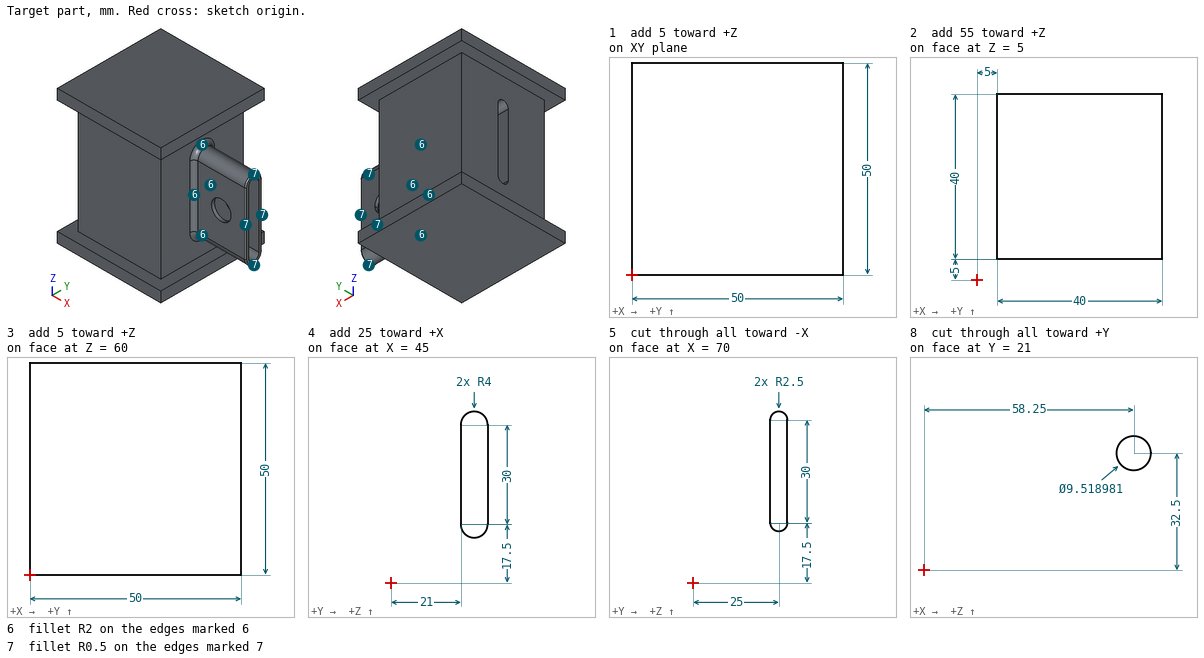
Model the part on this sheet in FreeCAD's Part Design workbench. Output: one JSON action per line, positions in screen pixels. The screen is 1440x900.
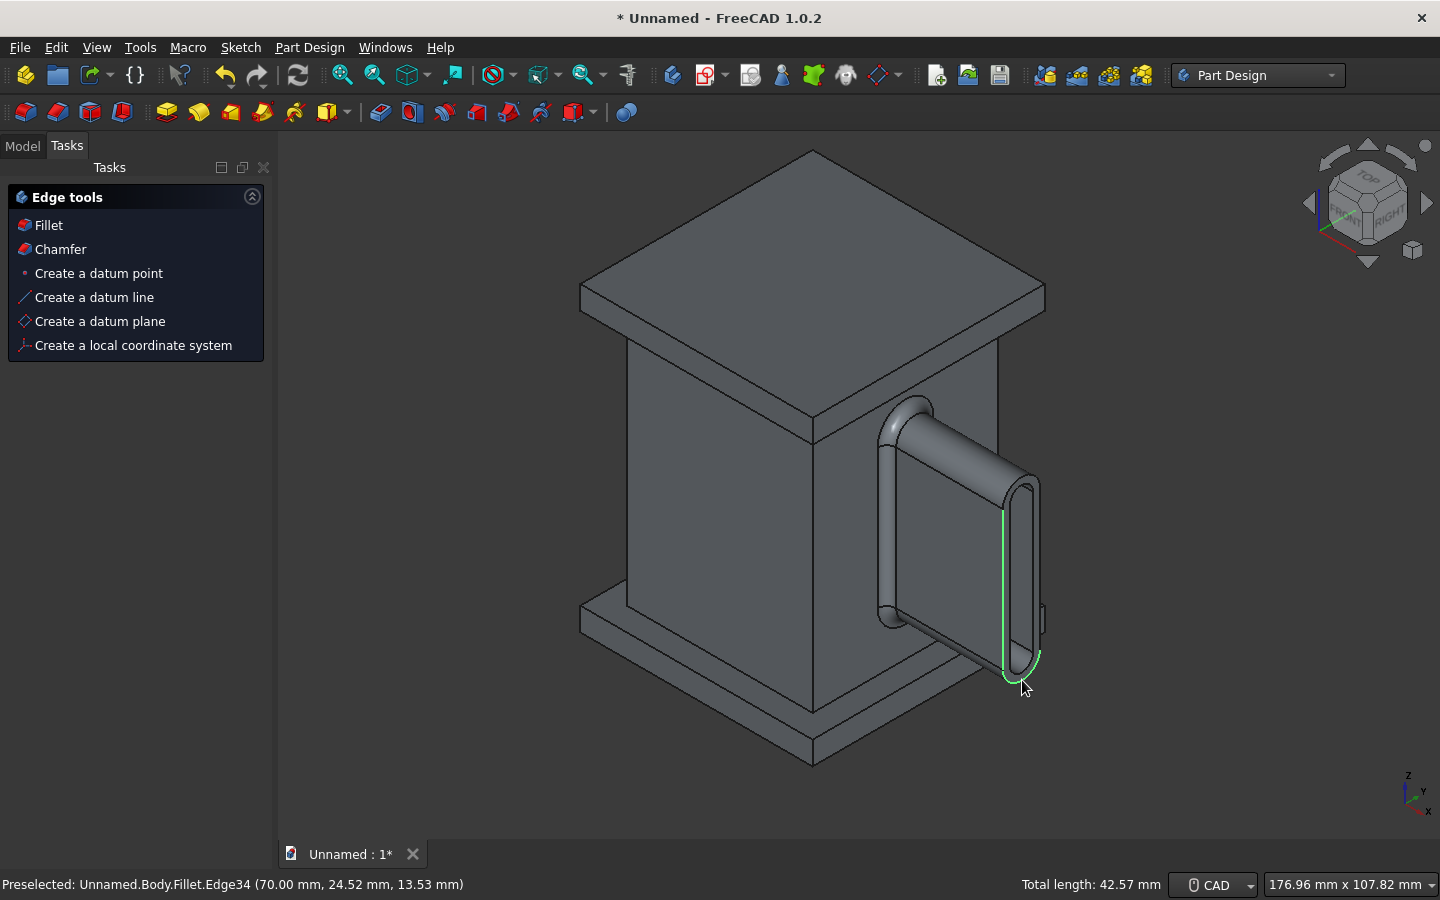
{"action": "left_click", "coordinate": [1022, 476], "text": "ctrl"}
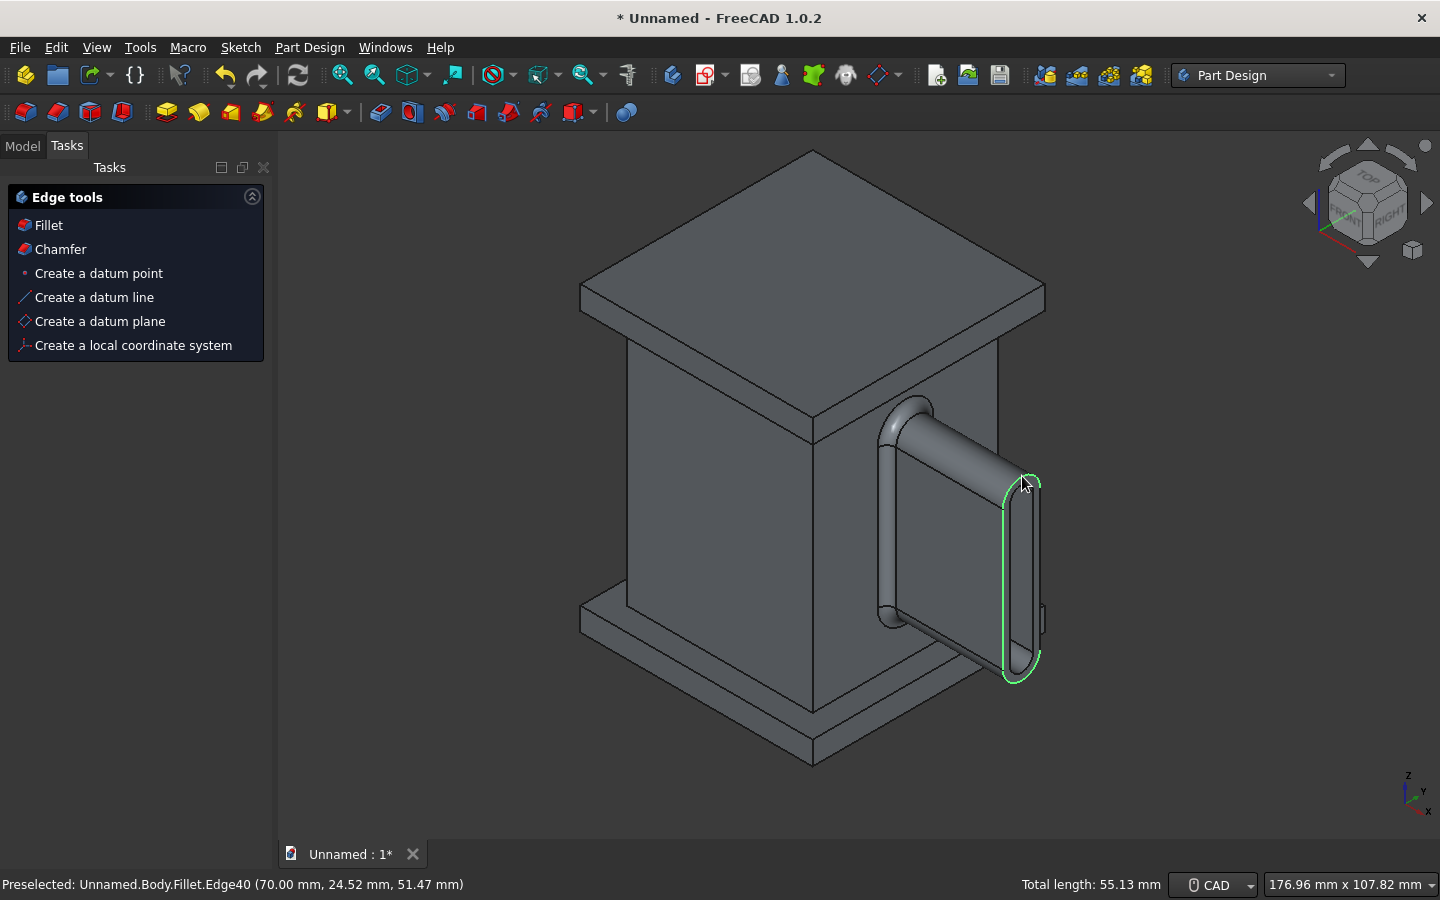
{"action": "key", "text": "2"}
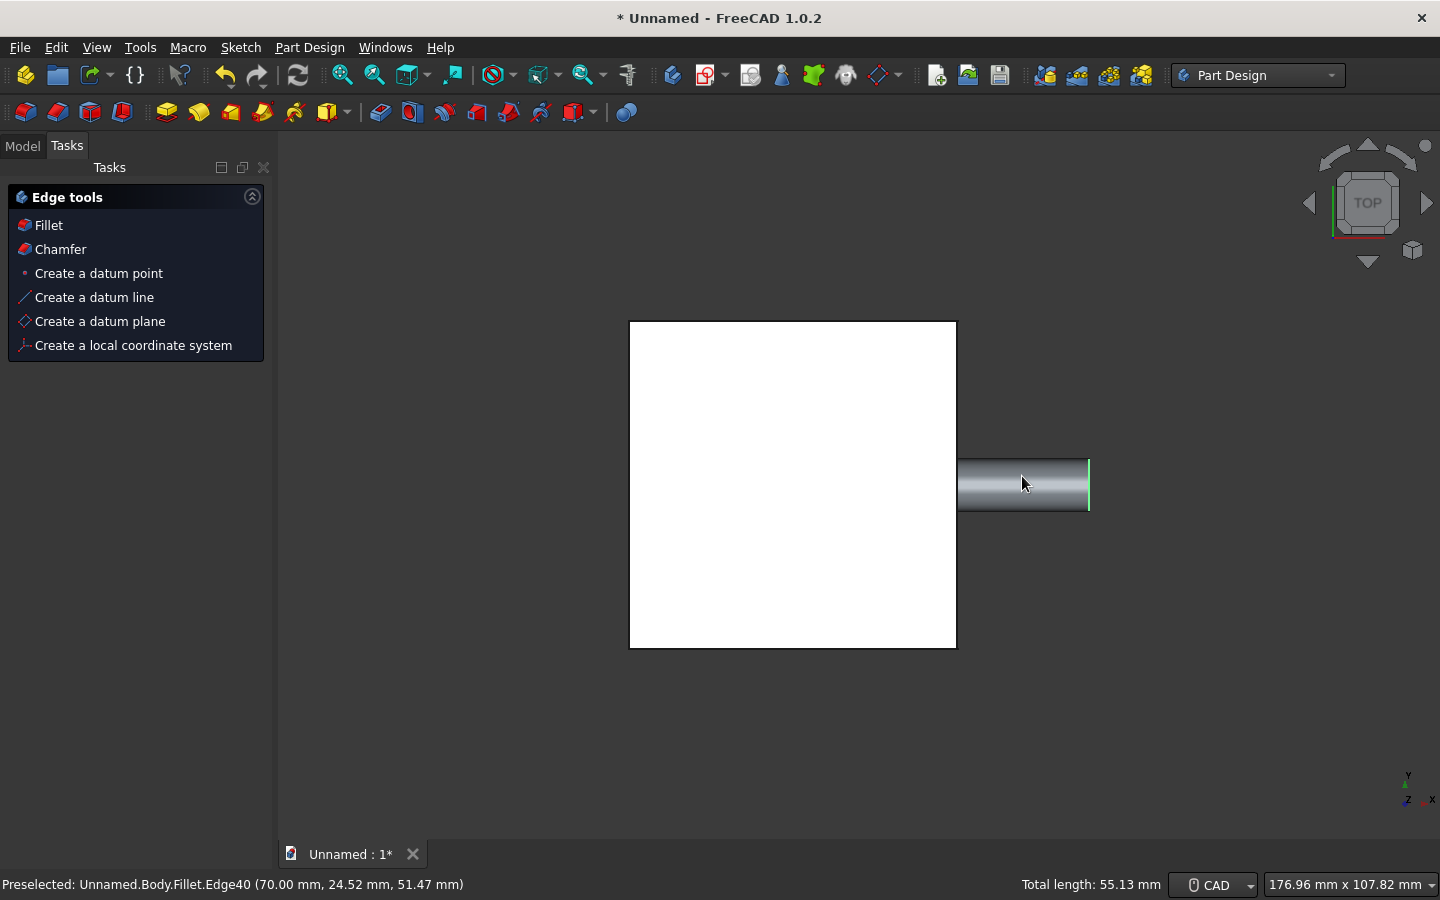
{"action": "key", "text": "0"}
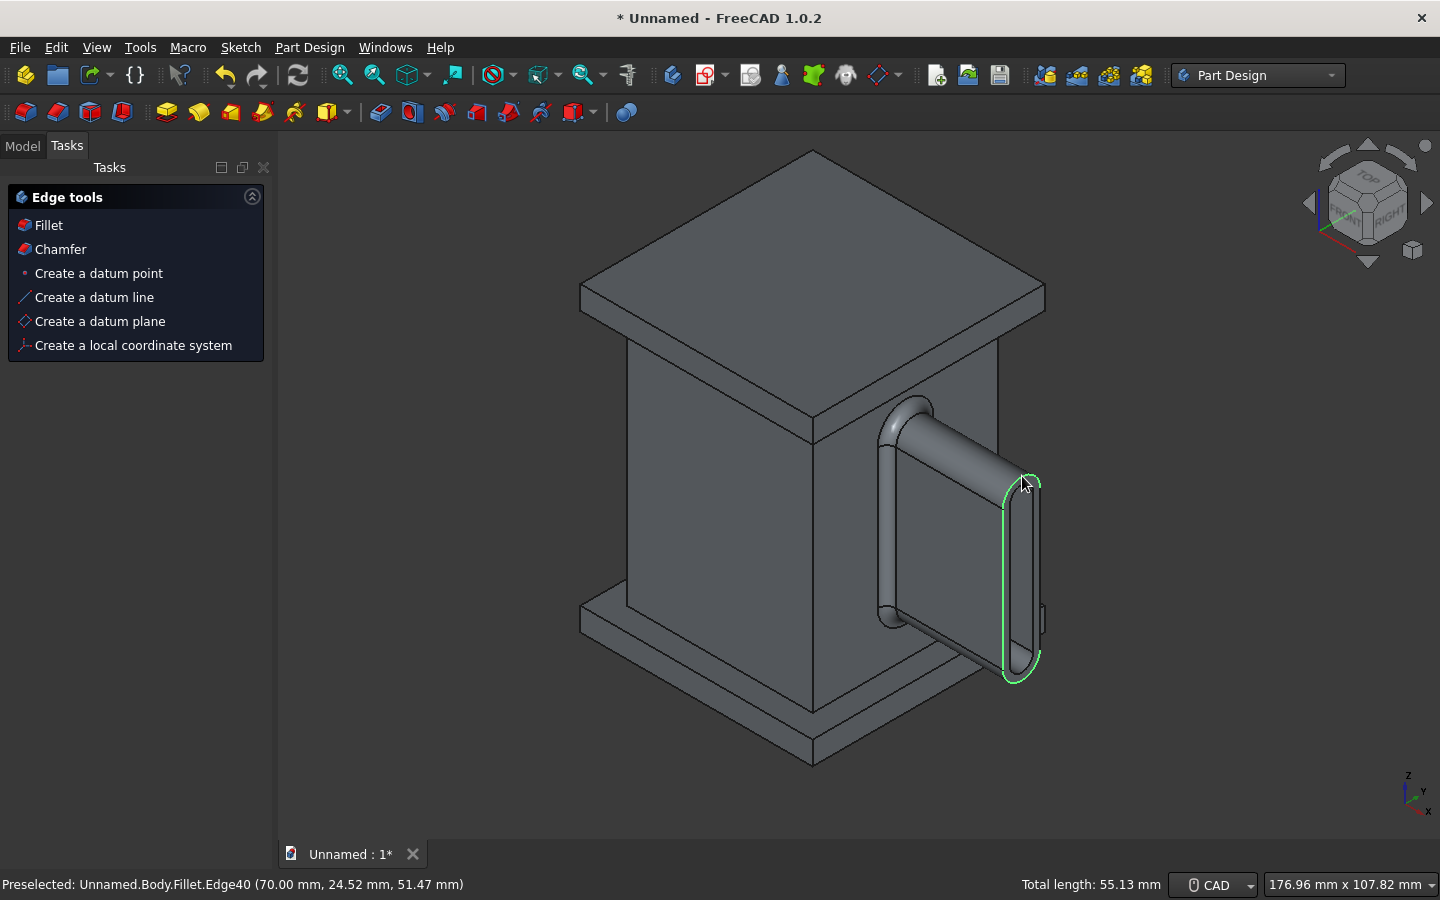
{"action": "key", "text": "1"}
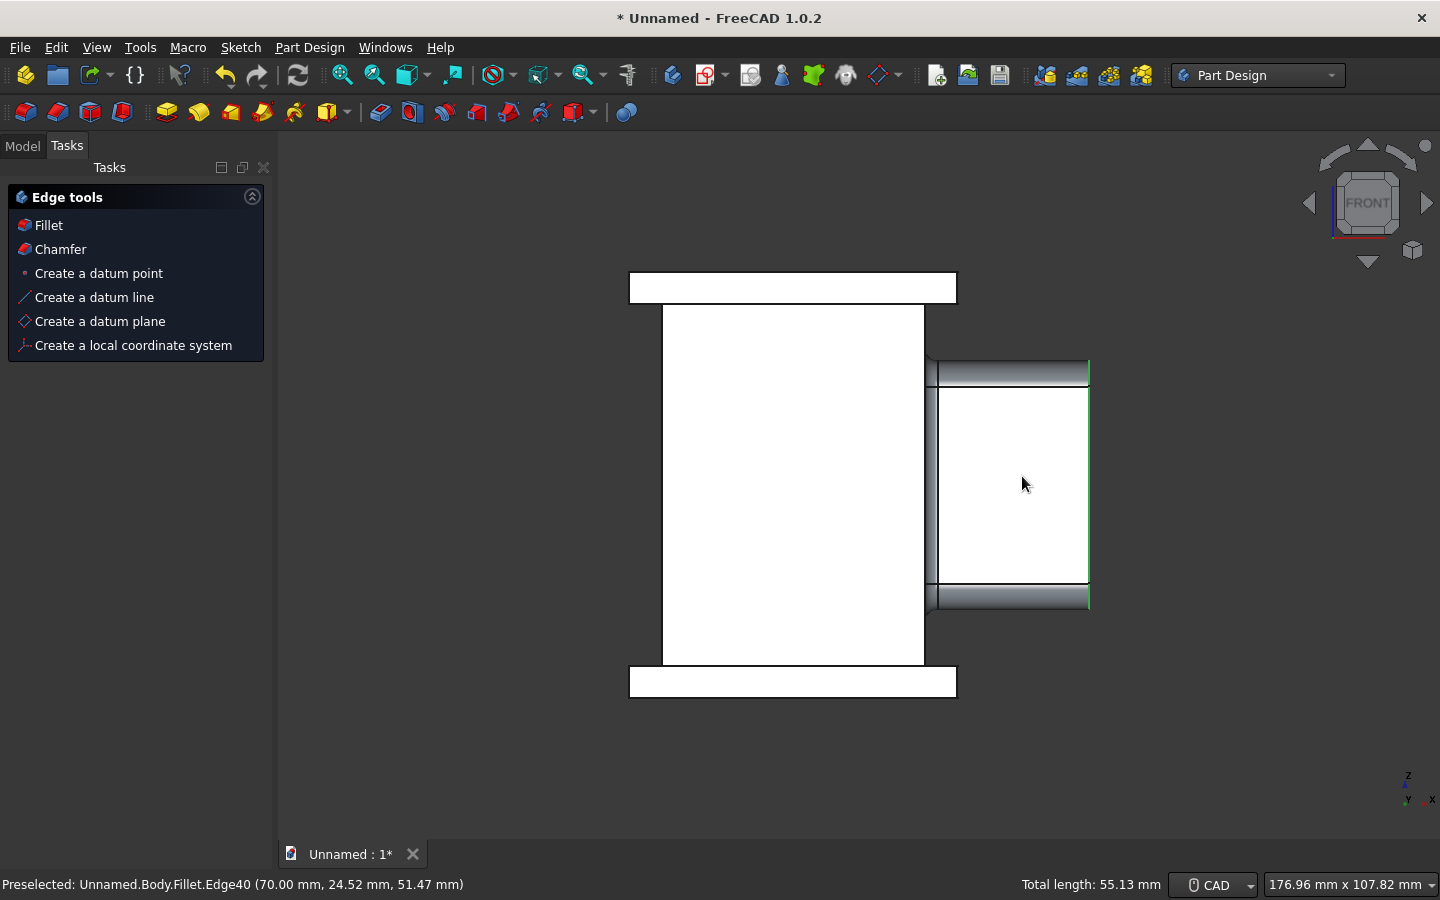
{"action": "key", "text": "3"}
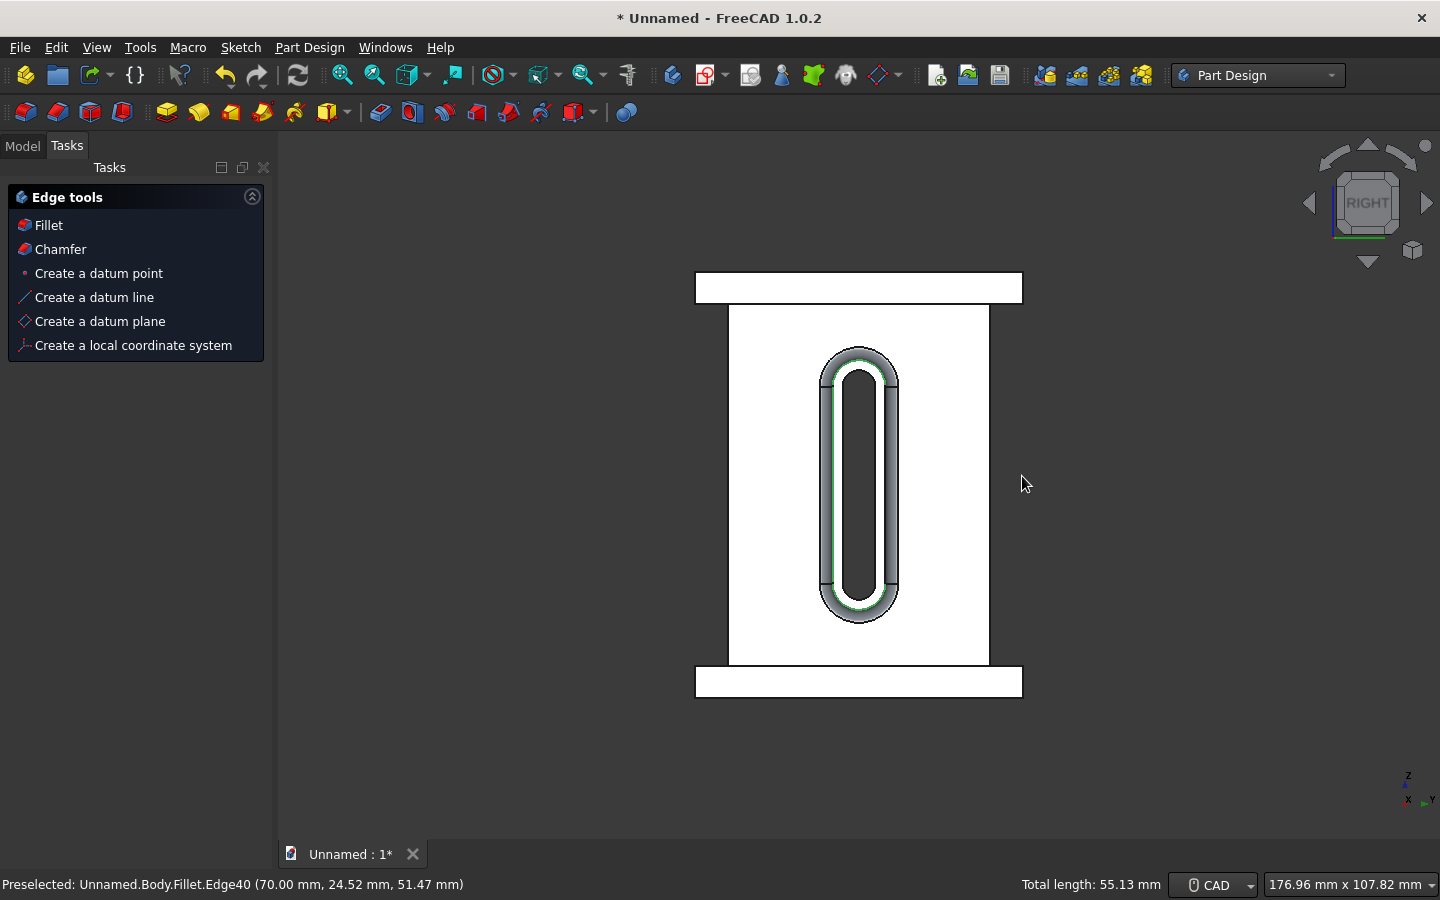
{"action": "left_click", "coordinate": [885, 484], "text": "ctrl"}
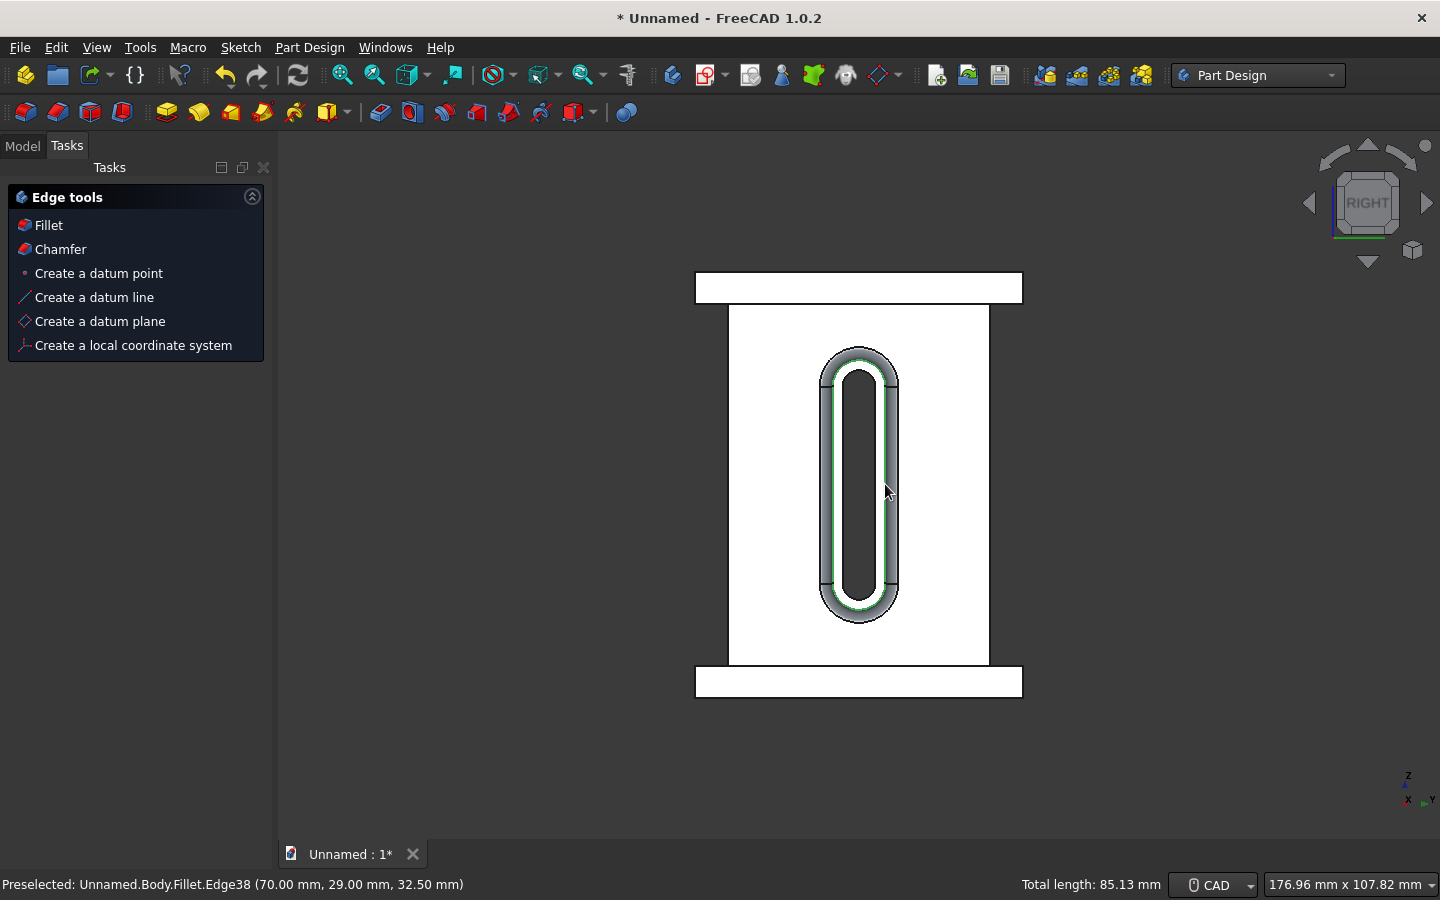
{"action": "left_click", "coordinate": [26, 112]}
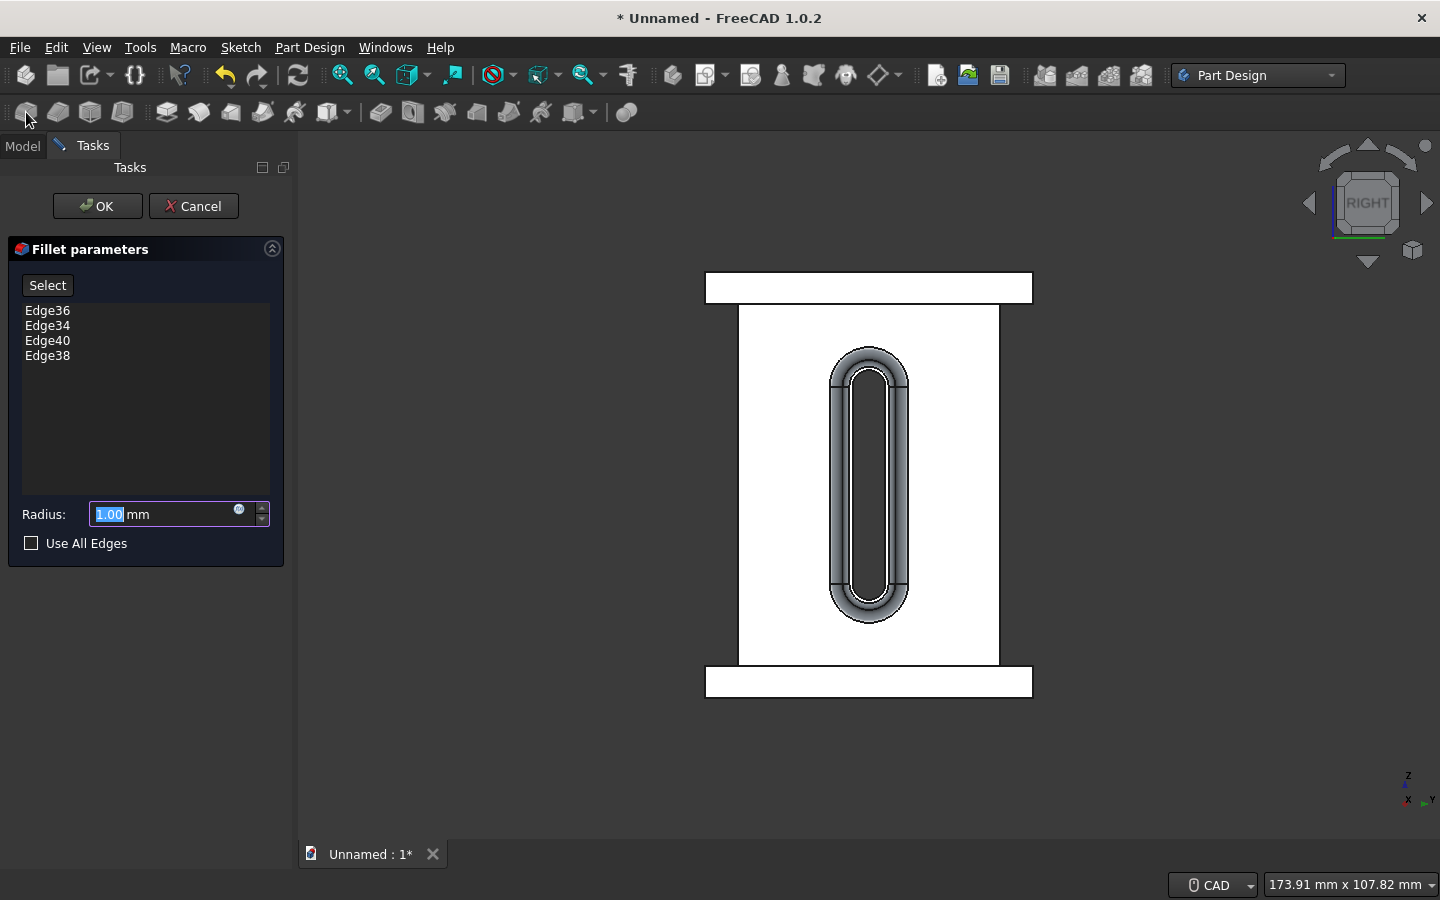
{"action": "type", "text": "0.5"}
{"action": "key", "text": "Tab"}